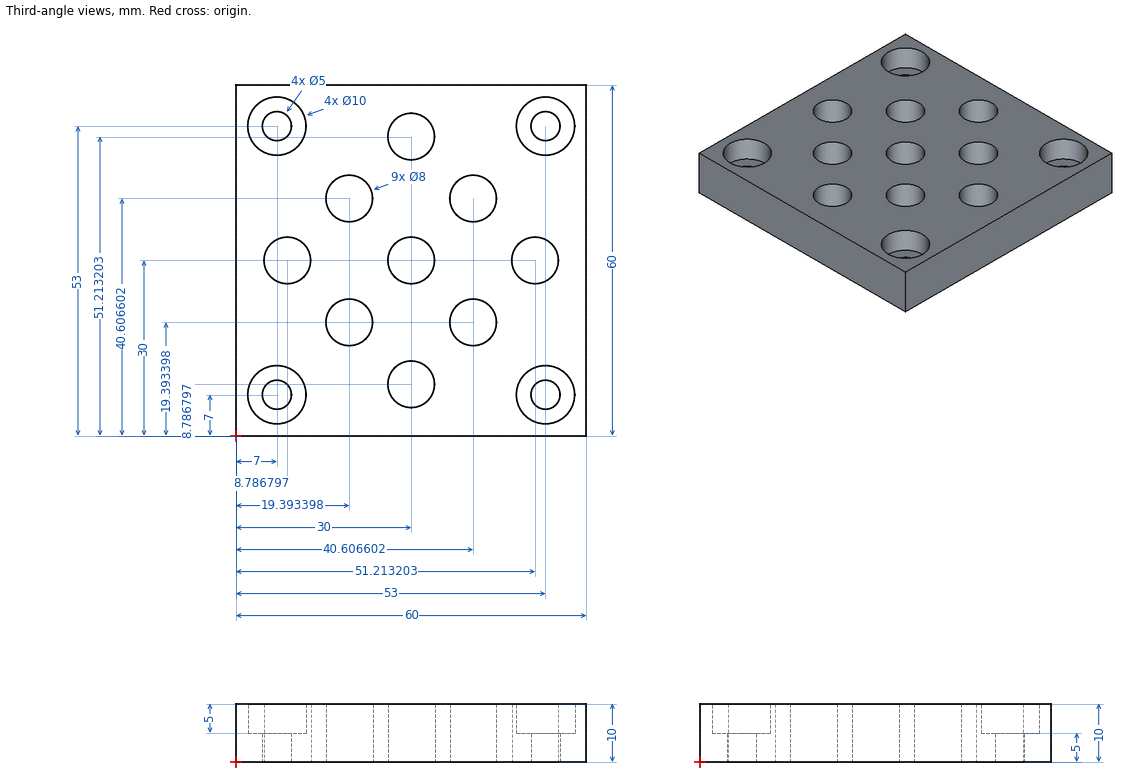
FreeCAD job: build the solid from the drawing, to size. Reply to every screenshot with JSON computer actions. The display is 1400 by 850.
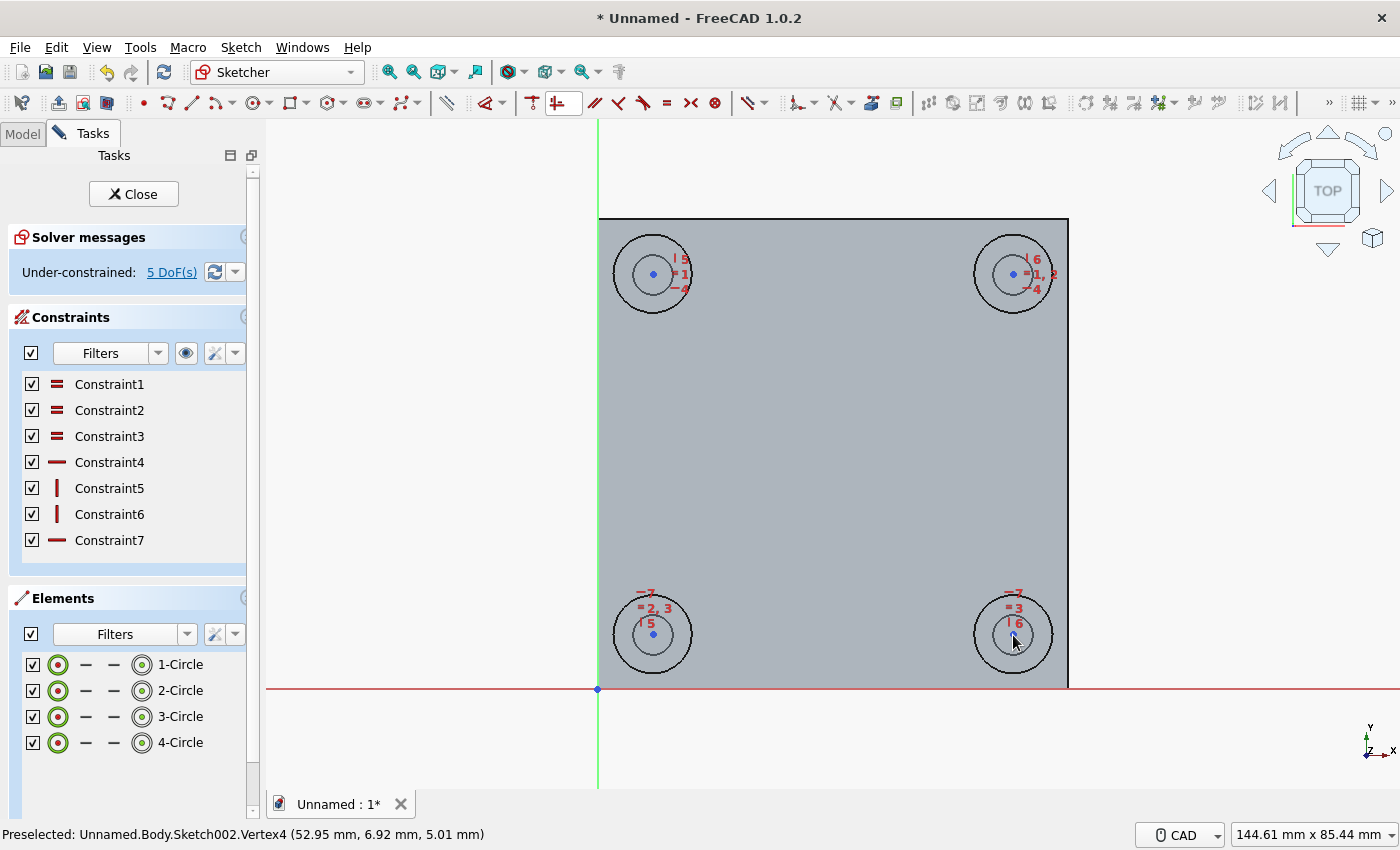
{"action": "key", "text": "d"}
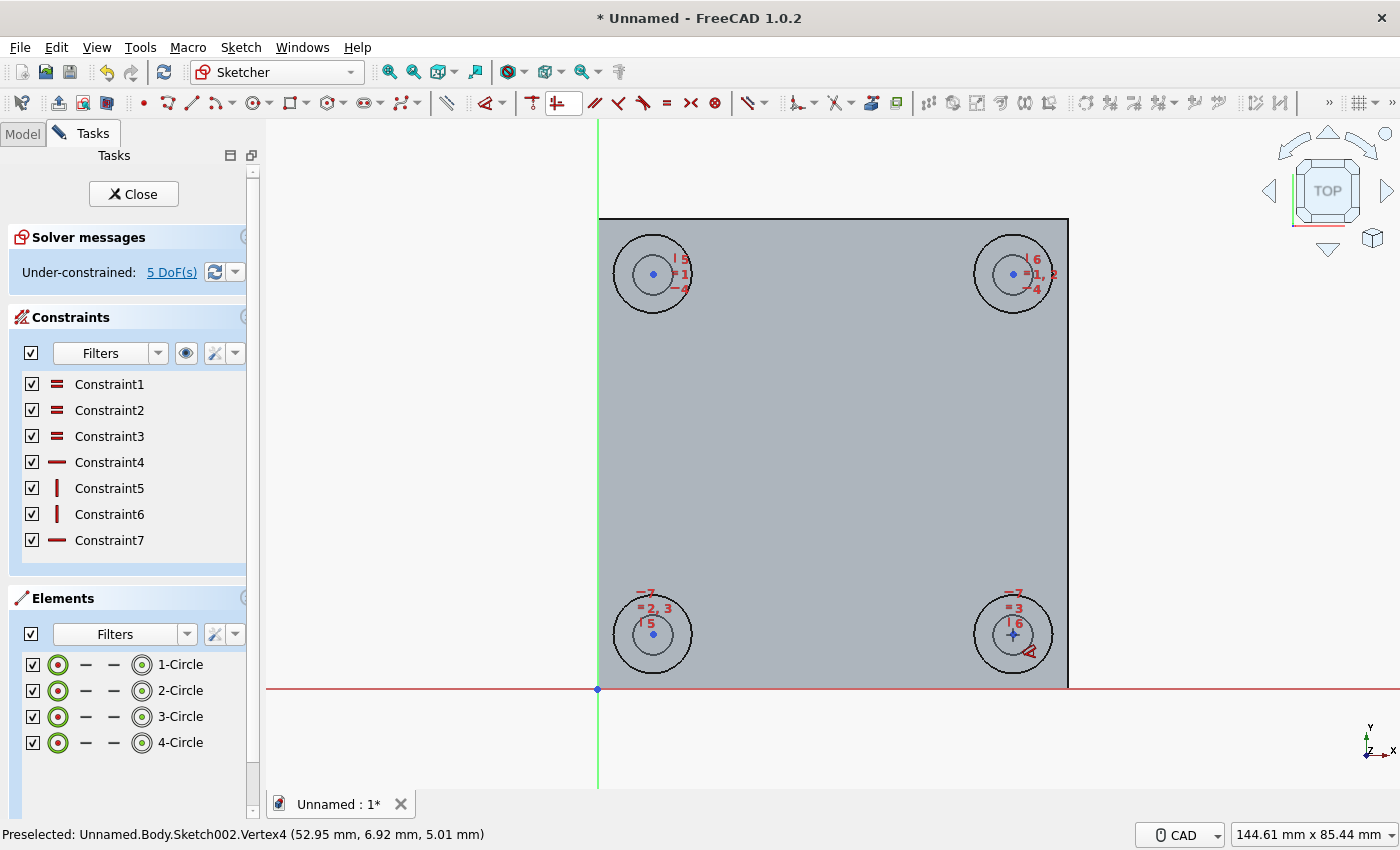
{"action": "left_click", "coordinate": [667, 261]}
{"action": "left_click", "coordinate": [690, 238]}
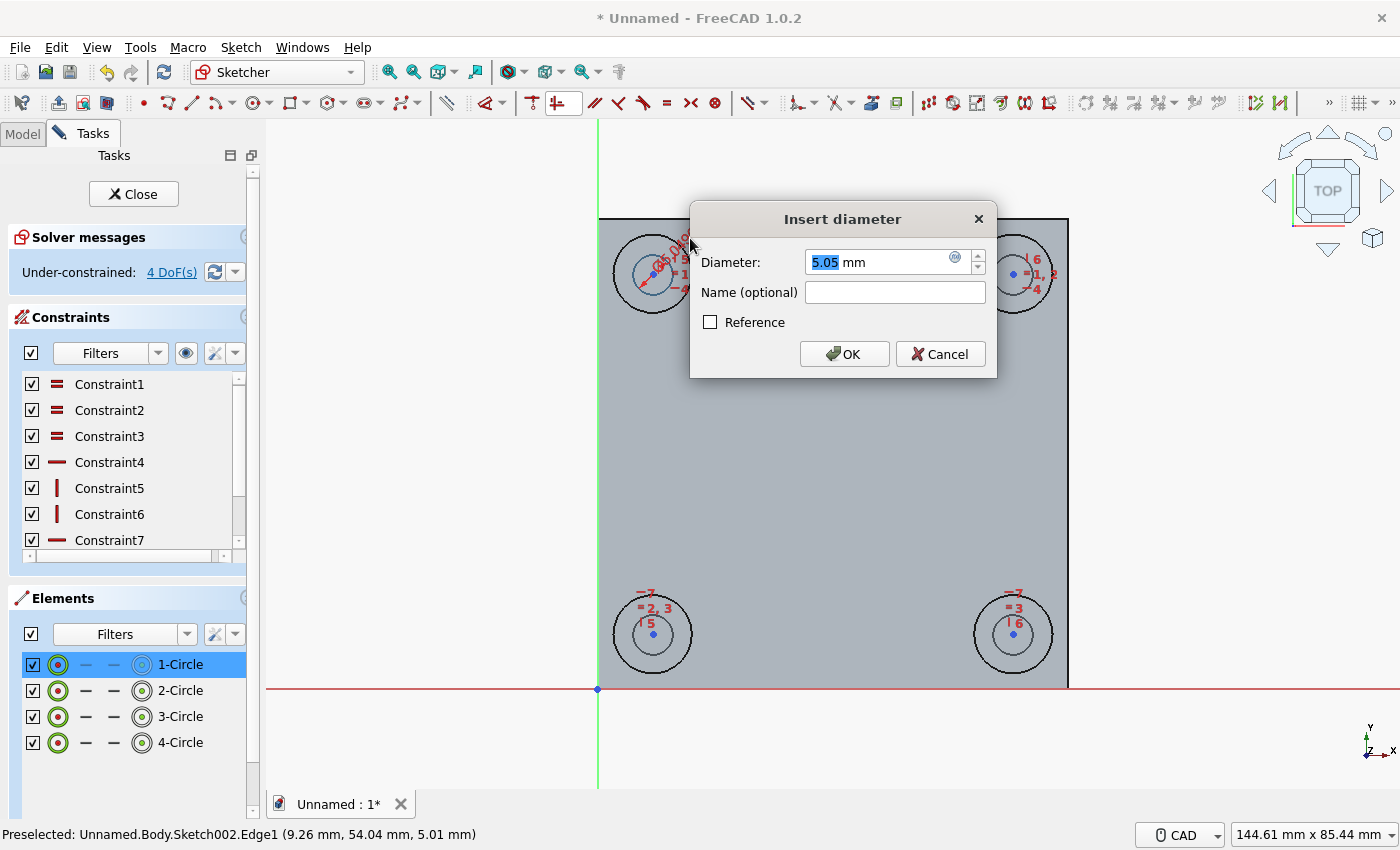
{"action": "type", "text": "5"}
{"action": "key", "text": "Return"}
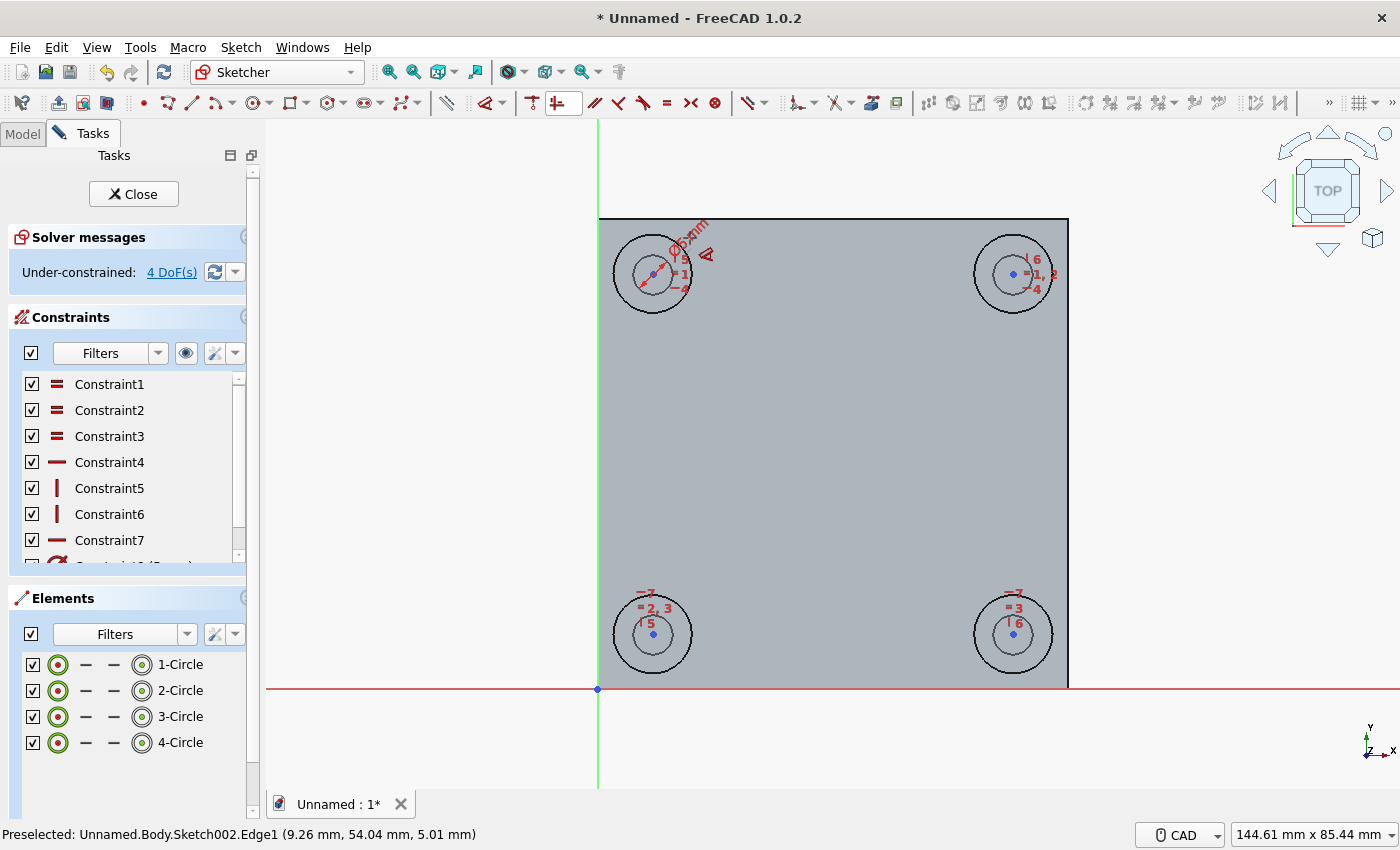
{"action": "left_click", "coordinate": [653, 275]}
{"action": "left_click", "coordinate": [625, 723]}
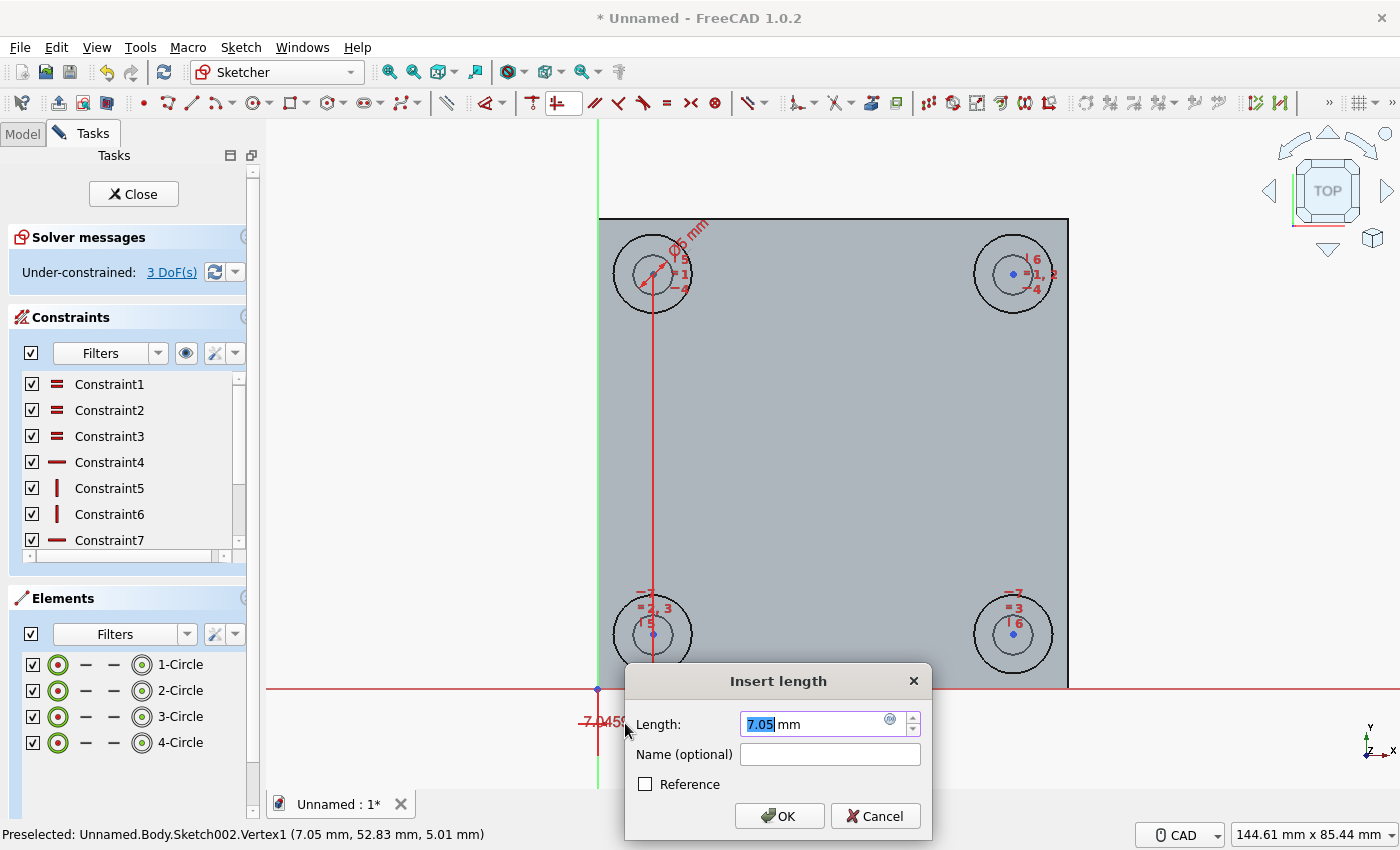
{"action": "type", "text": "7"}
{"action": "key", "text": "Return"}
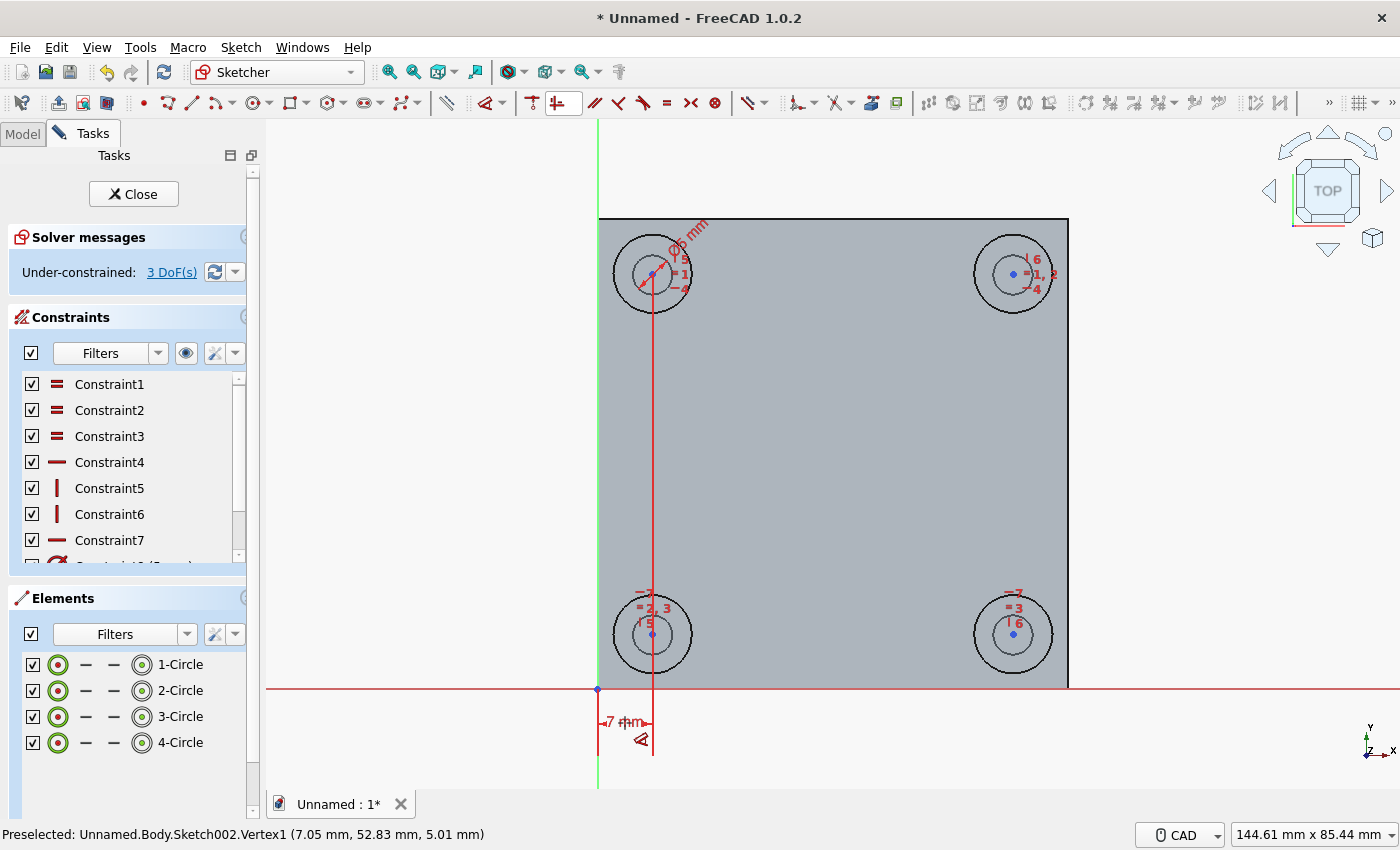
{"action": "left_click", "coordinate": [653, 635]}
{"action": "left_click", "coordinate": [564, 662]}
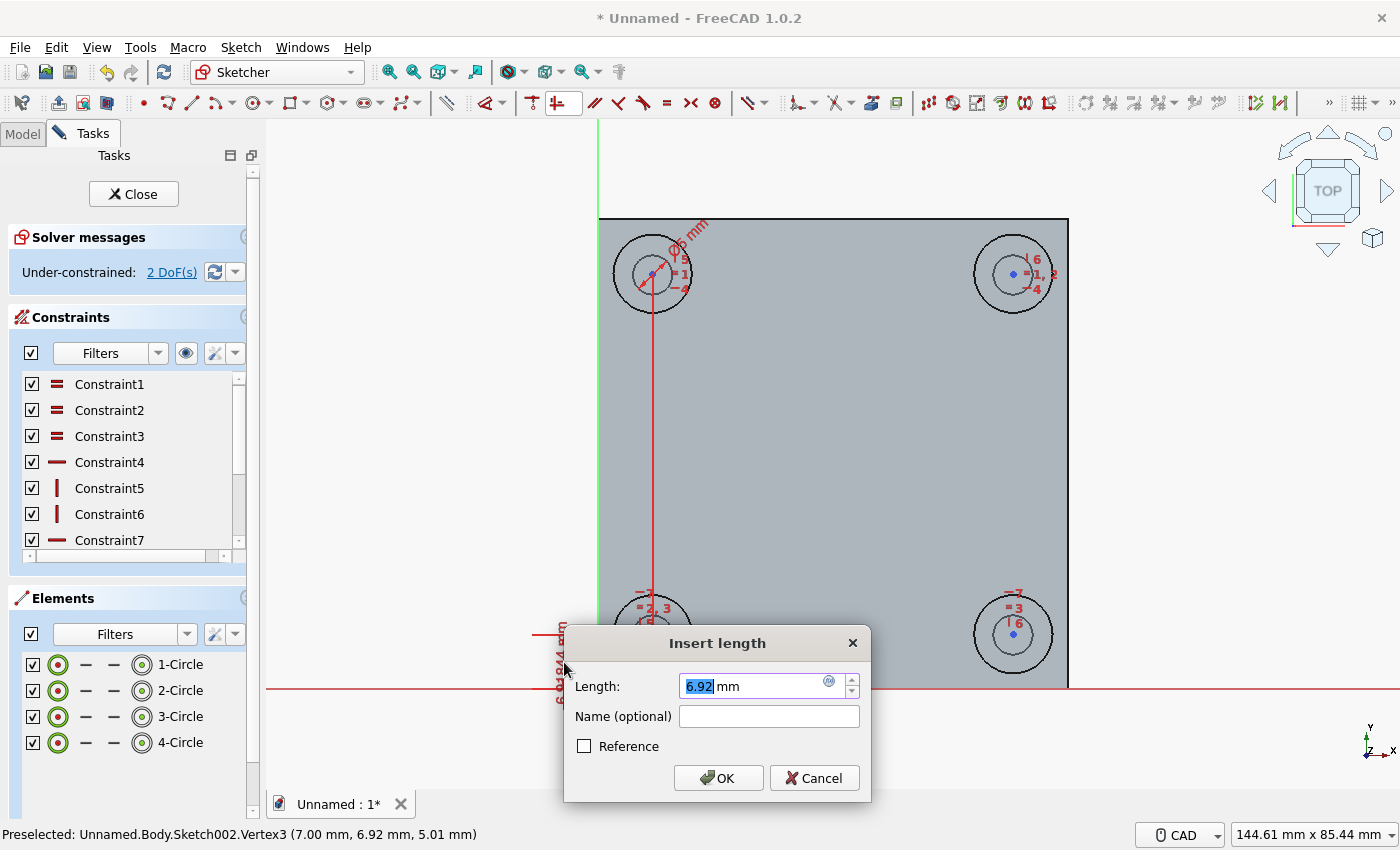
{"action": "type", "text": "7"}
{"action": "key", "text": "Return"}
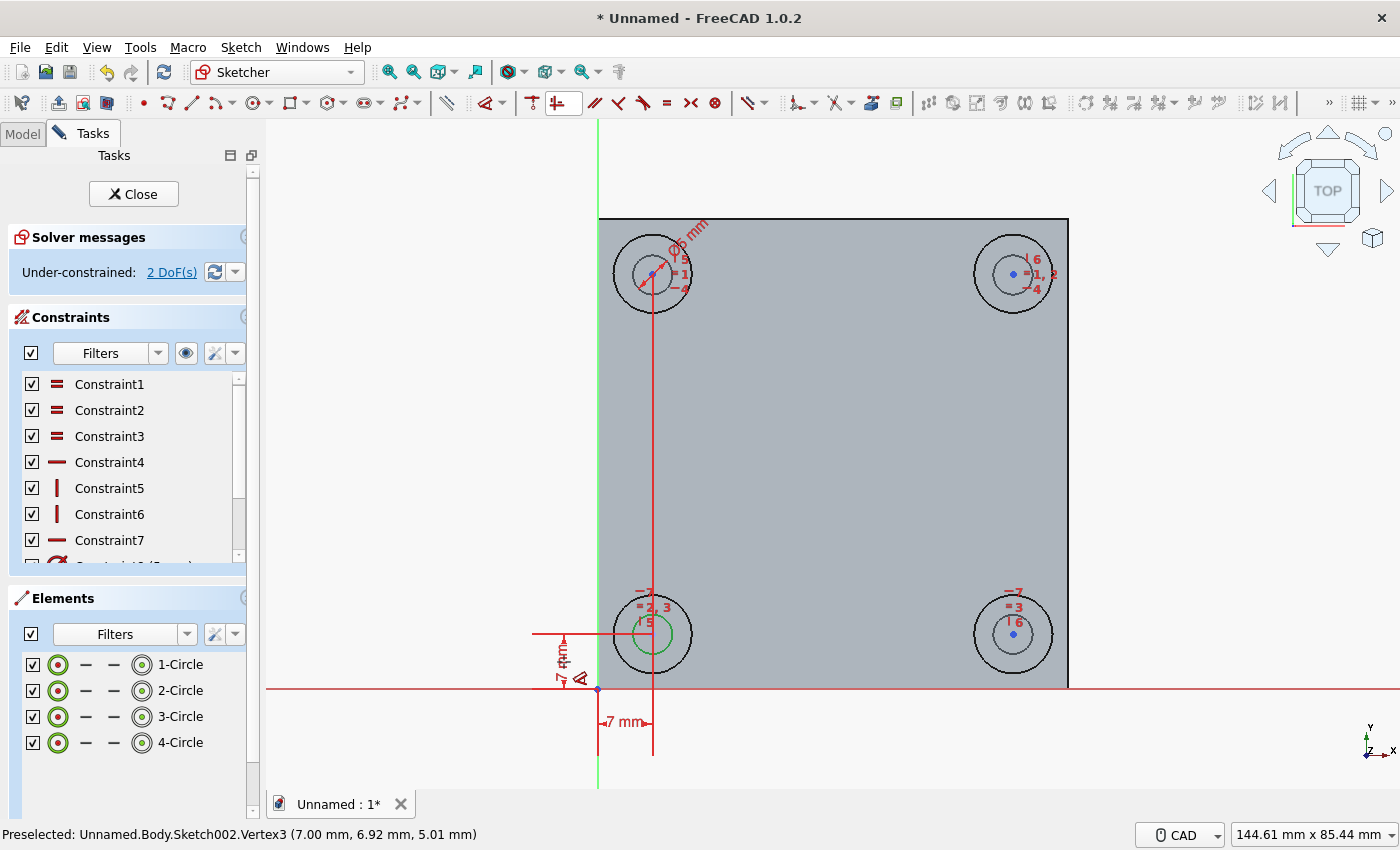
{"action": "left_click", "coordinate": [653, 275]}
{"action": "left_click", "coordinate": [564, 482]}